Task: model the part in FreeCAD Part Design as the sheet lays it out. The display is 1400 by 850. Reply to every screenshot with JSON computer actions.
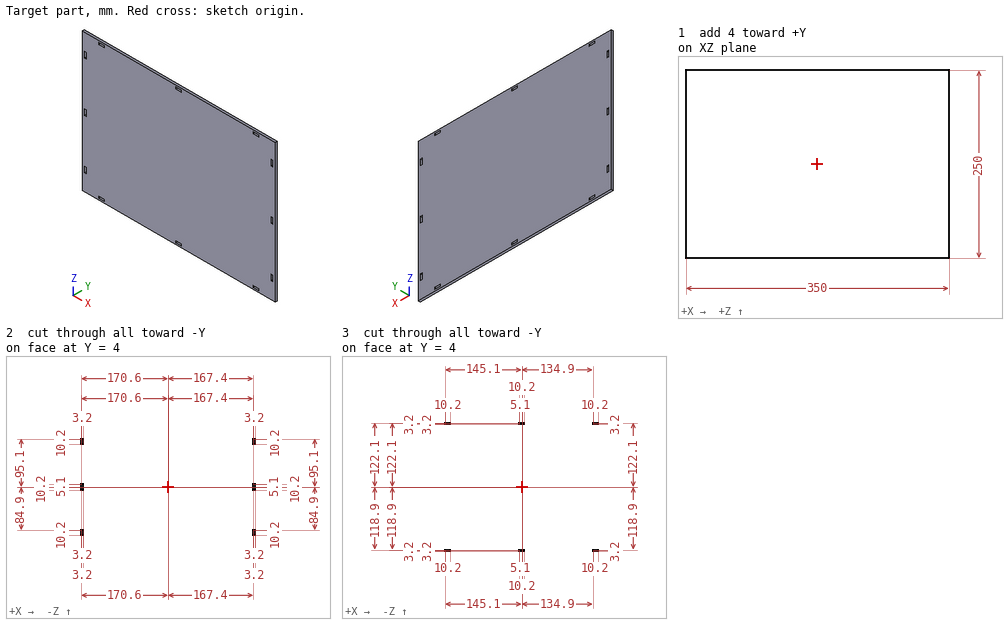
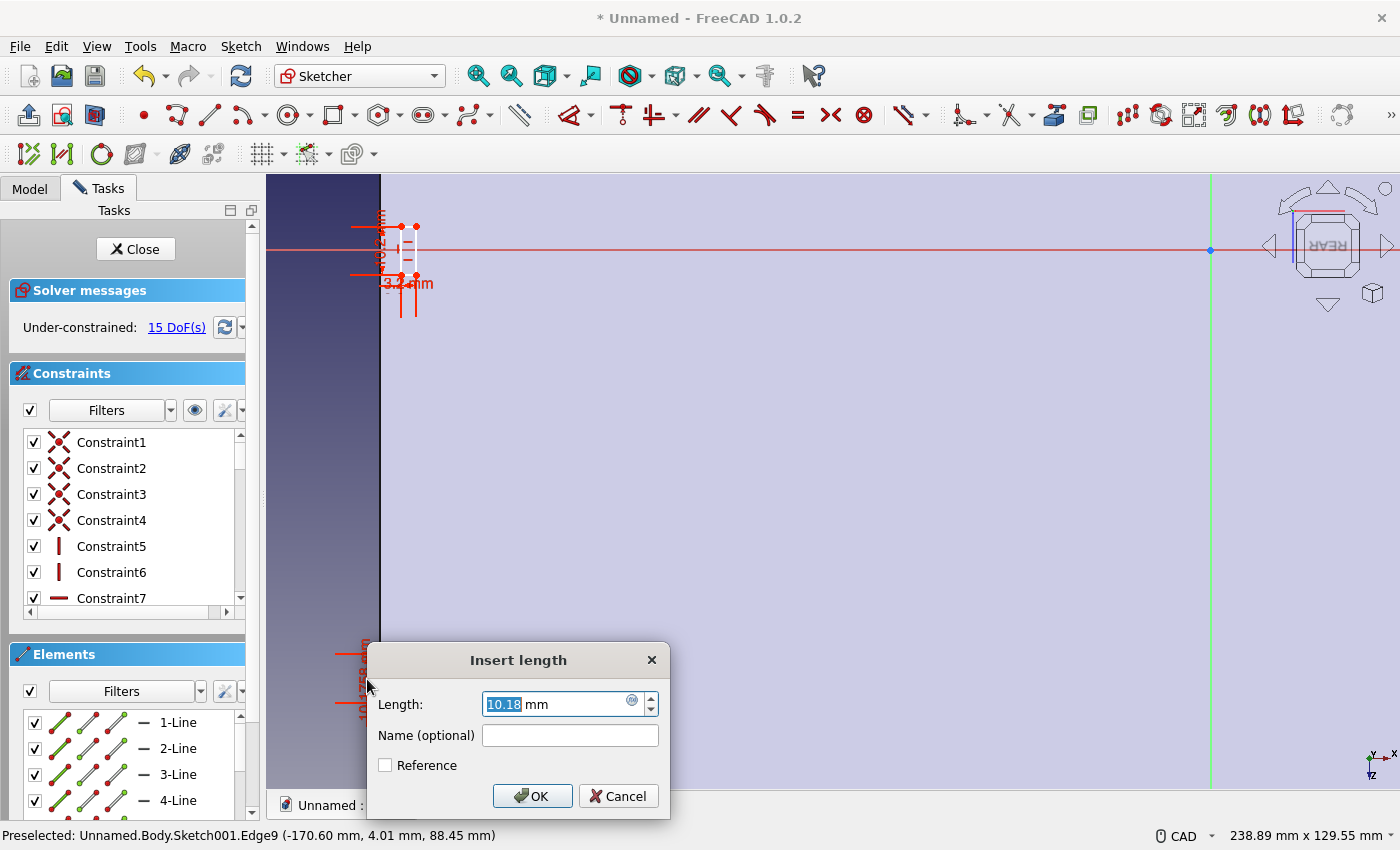
{"action": "type", "text": "10.2"}
{"action": "key", "text": "Return"}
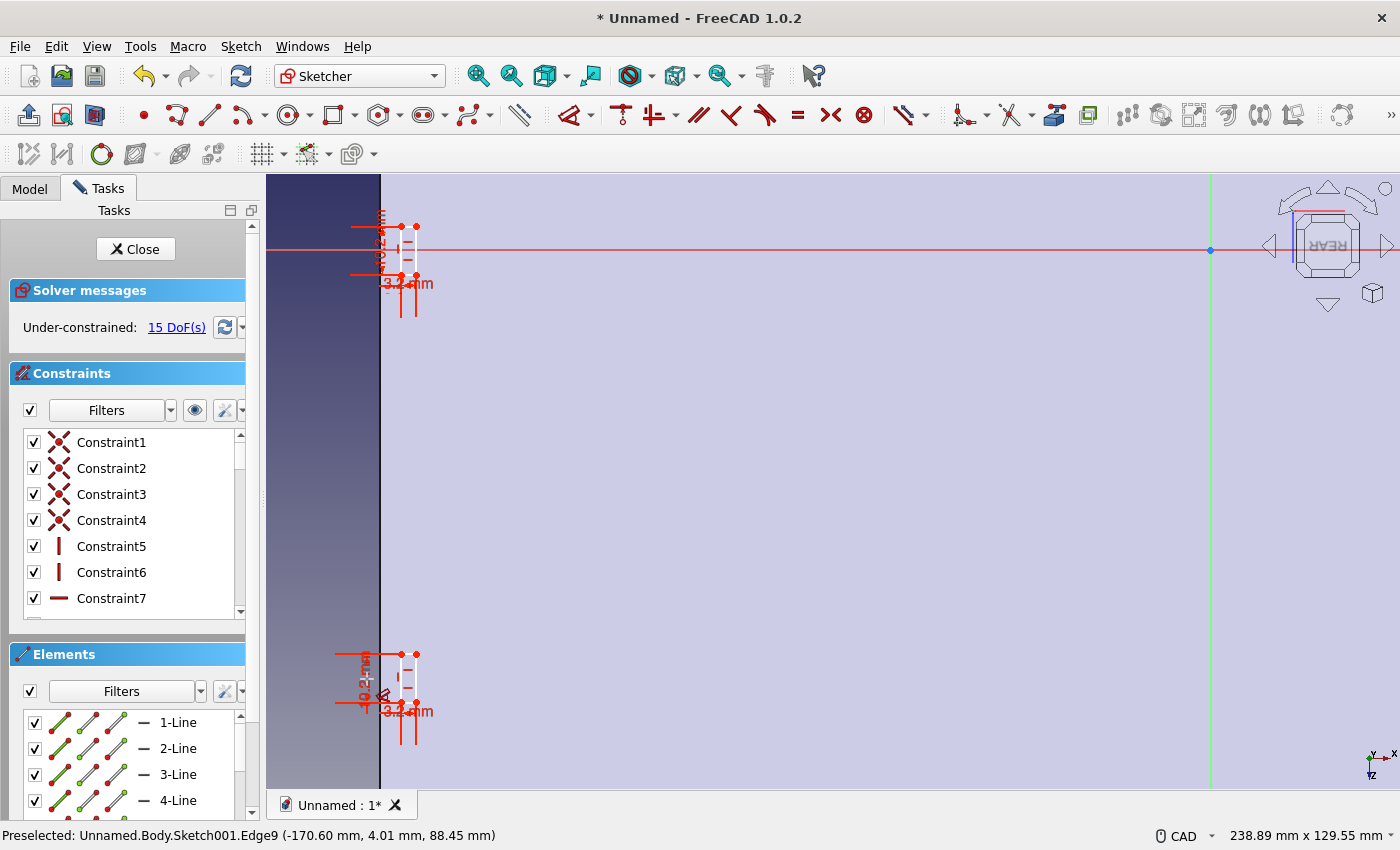
{"action": "scroll", "coordinate": [400, 670], "scroll_direction": "down", "scroll_amount": 4}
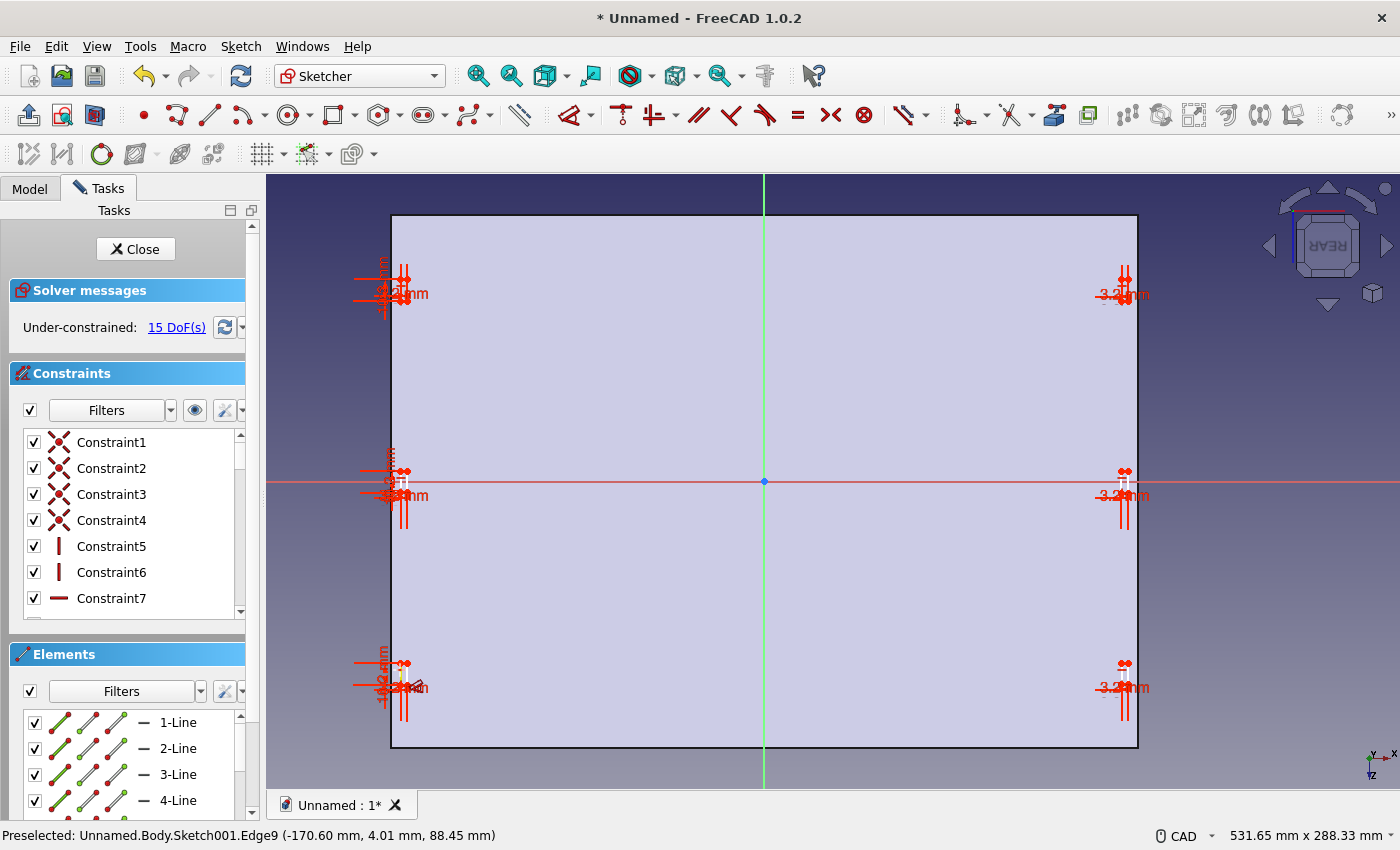
{"action": "scroll", "coordinate": [1122, 670], "scroll_direction": "up", "scroll_amount": 4}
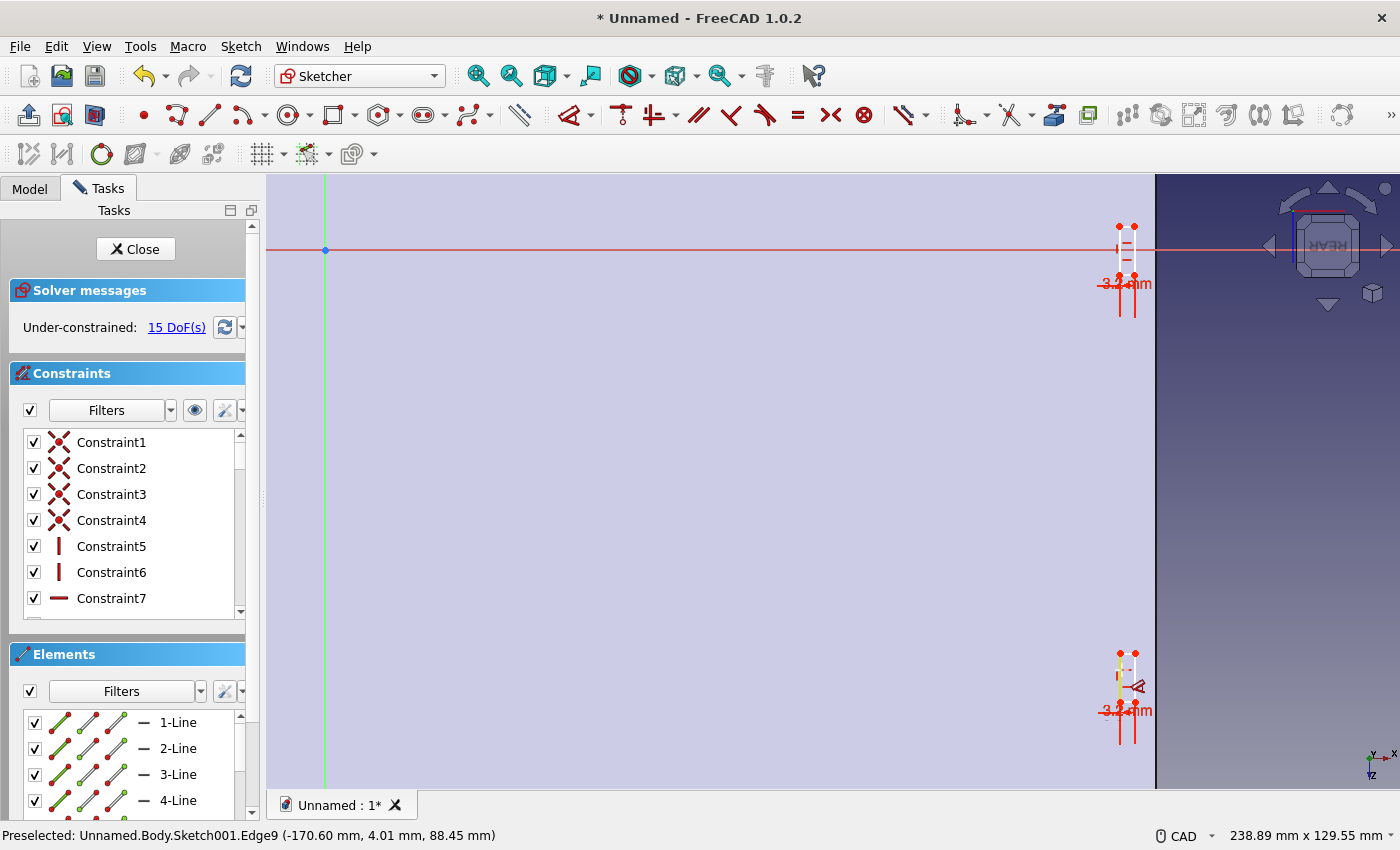
{"action": "left_click", "coordinate": [1120, 668]}
{"action": "left_click", "coordinate": [1154, 678]}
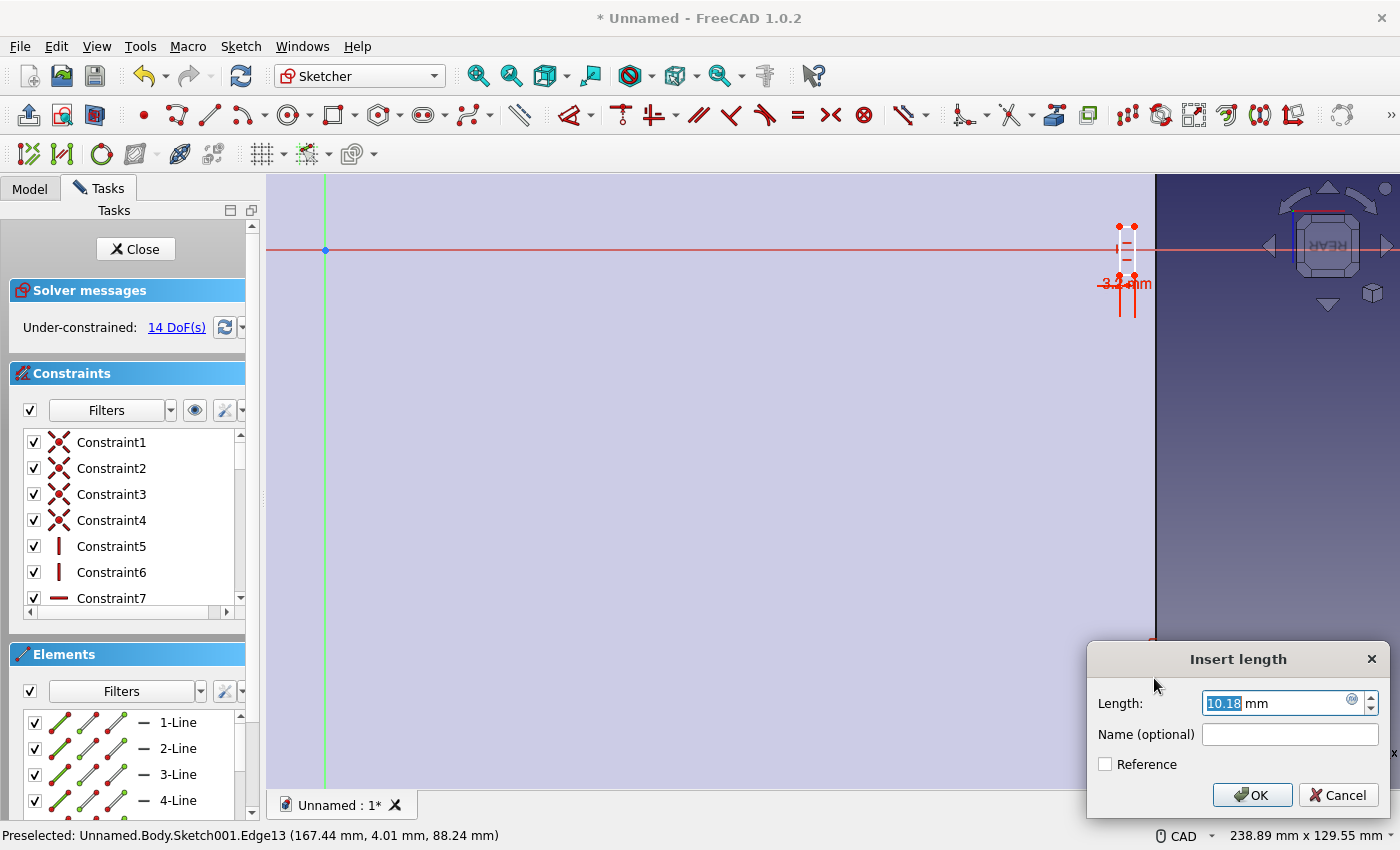
{"action": "type", "text": "10.2"}
{"action": "key", "text": "Return"}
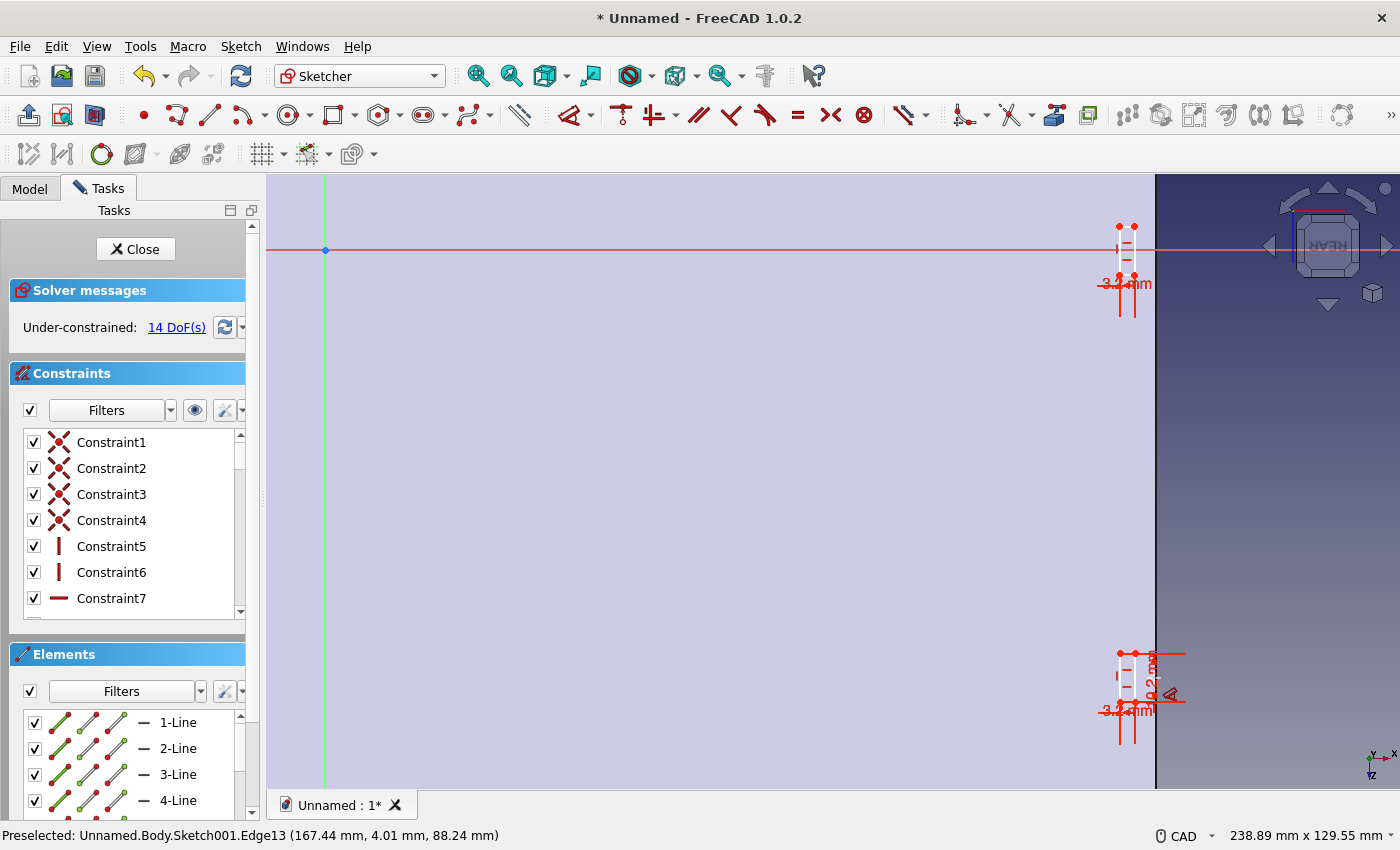
{"action": "scroll", "coordinate": [1120, 261], "scroll_direction": "up", "scroll_amount": 2}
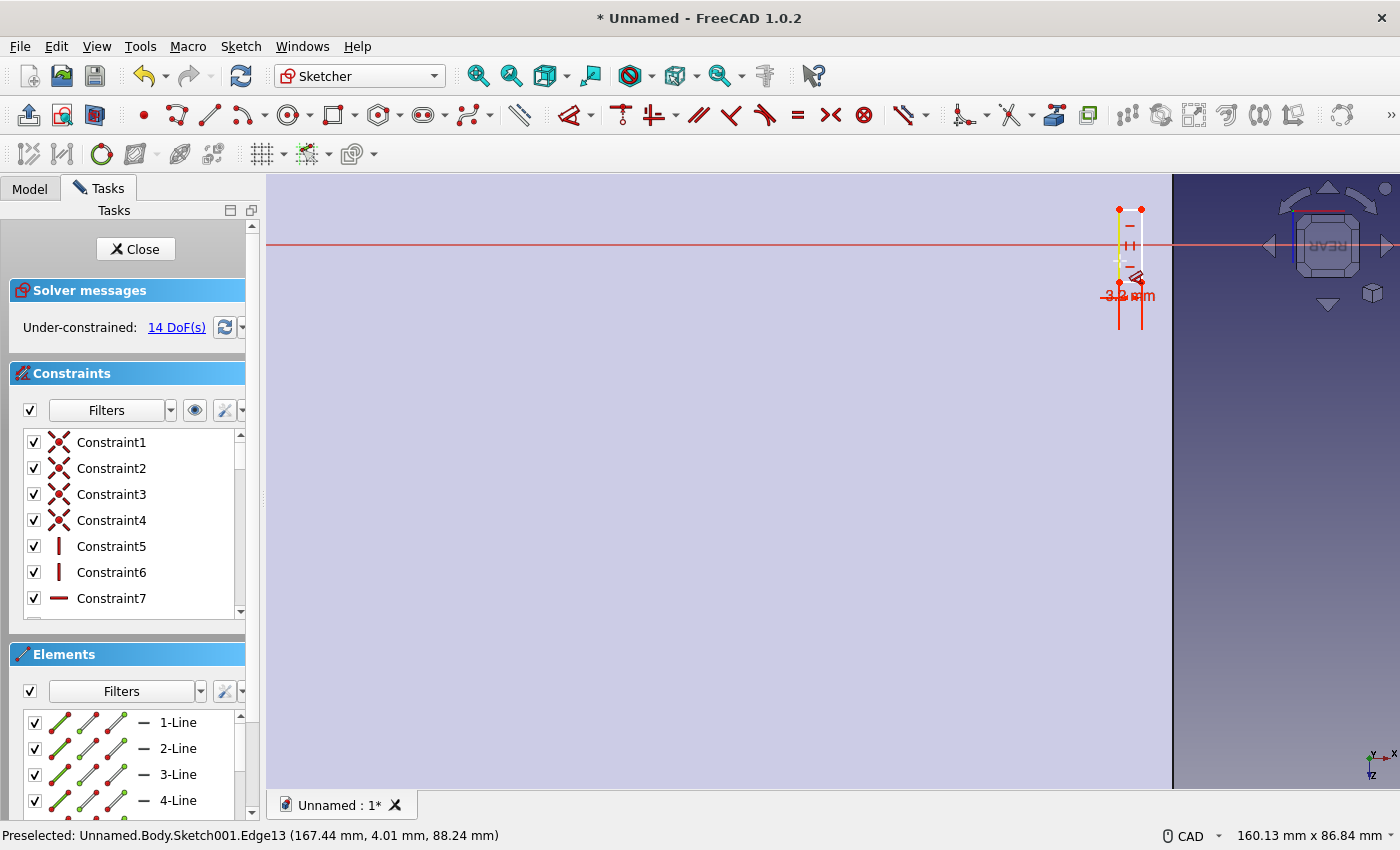
{"action": "left_click", "coordinate": [1119, 260]}
{"action": "left_click", "coordinate": [1085, 229]}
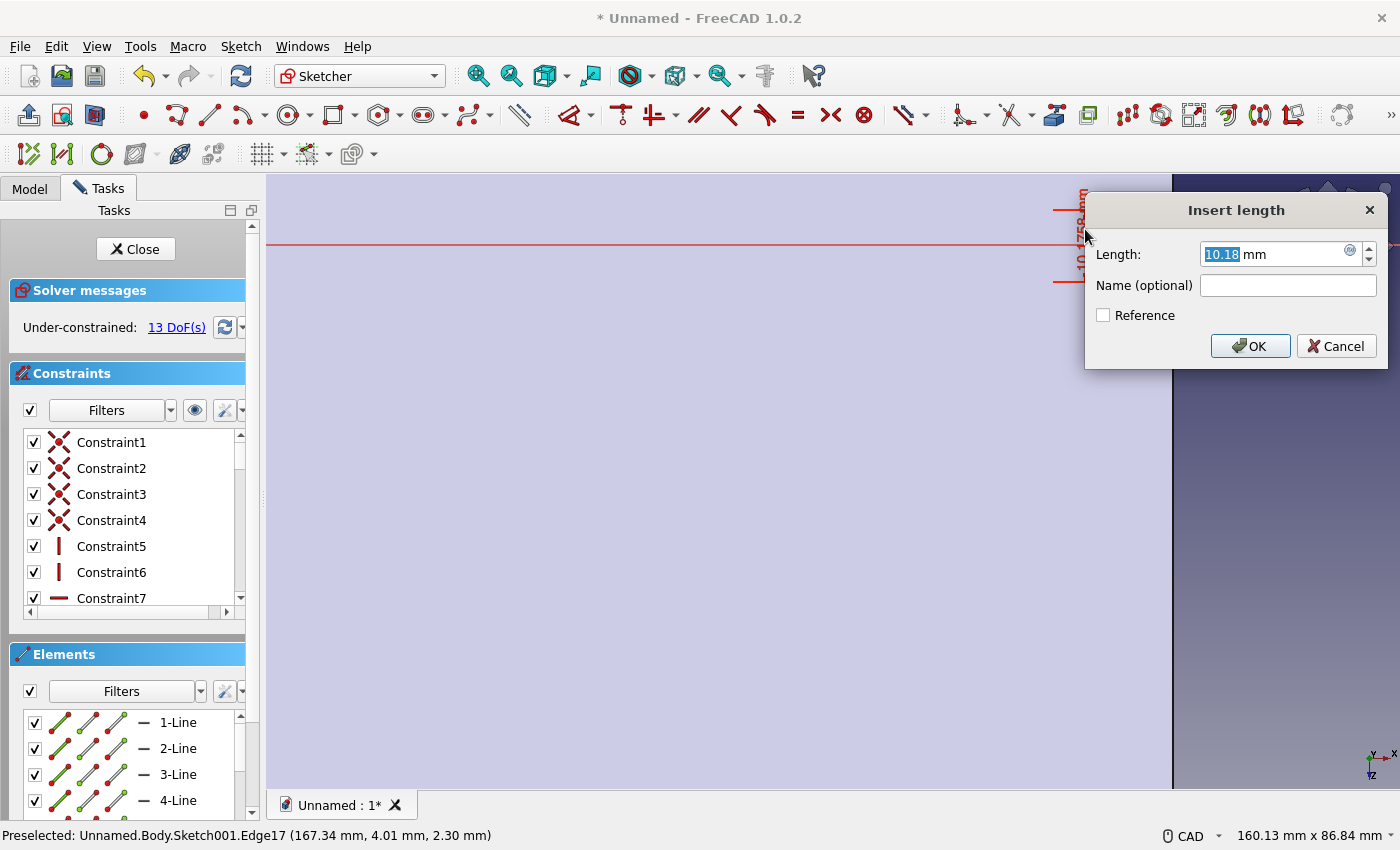
{"action": "type", "text": "10.2"}
{"action": "key", "text": "Return"}